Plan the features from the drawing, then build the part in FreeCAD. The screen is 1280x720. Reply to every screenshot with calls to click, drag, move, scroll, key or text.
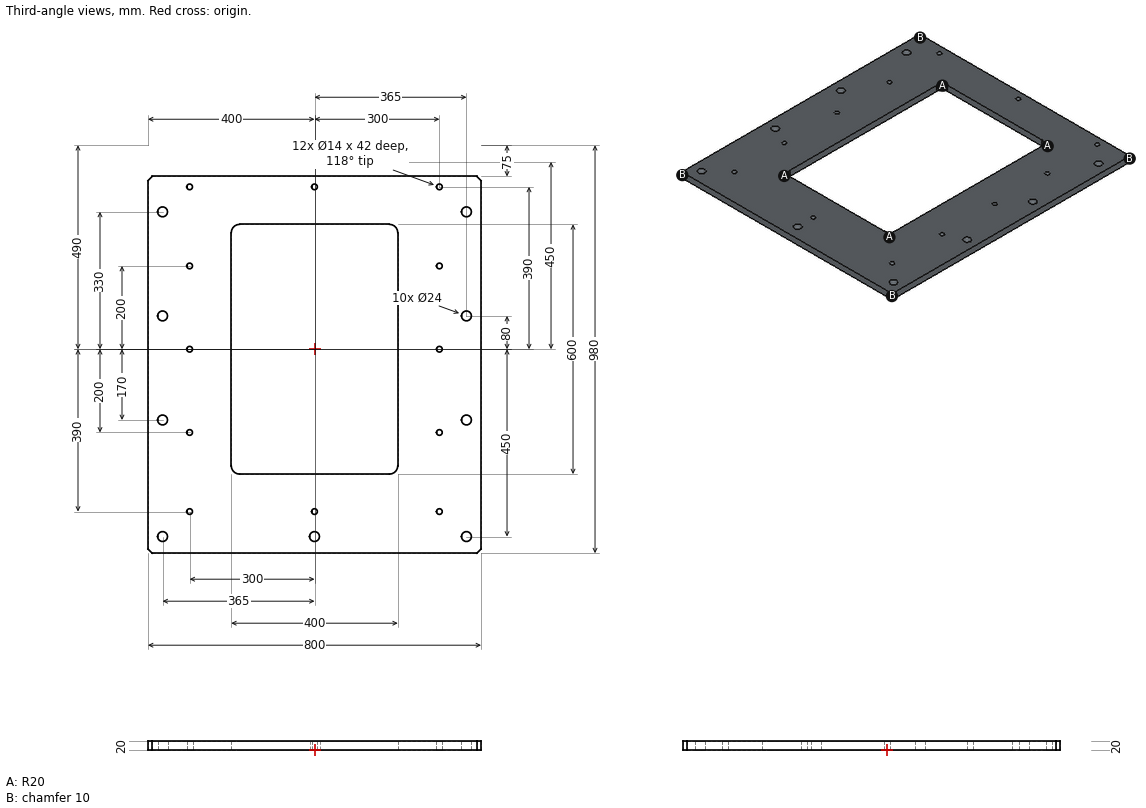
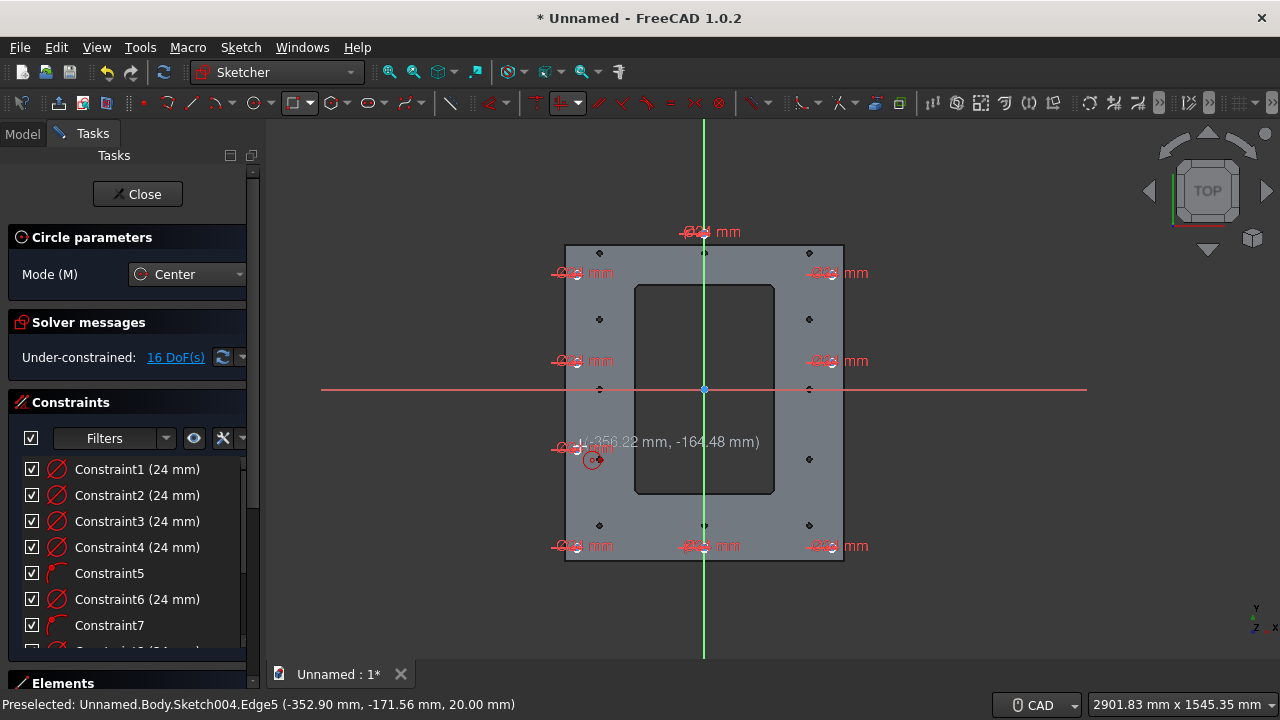
scroll(832, 449, up, 9)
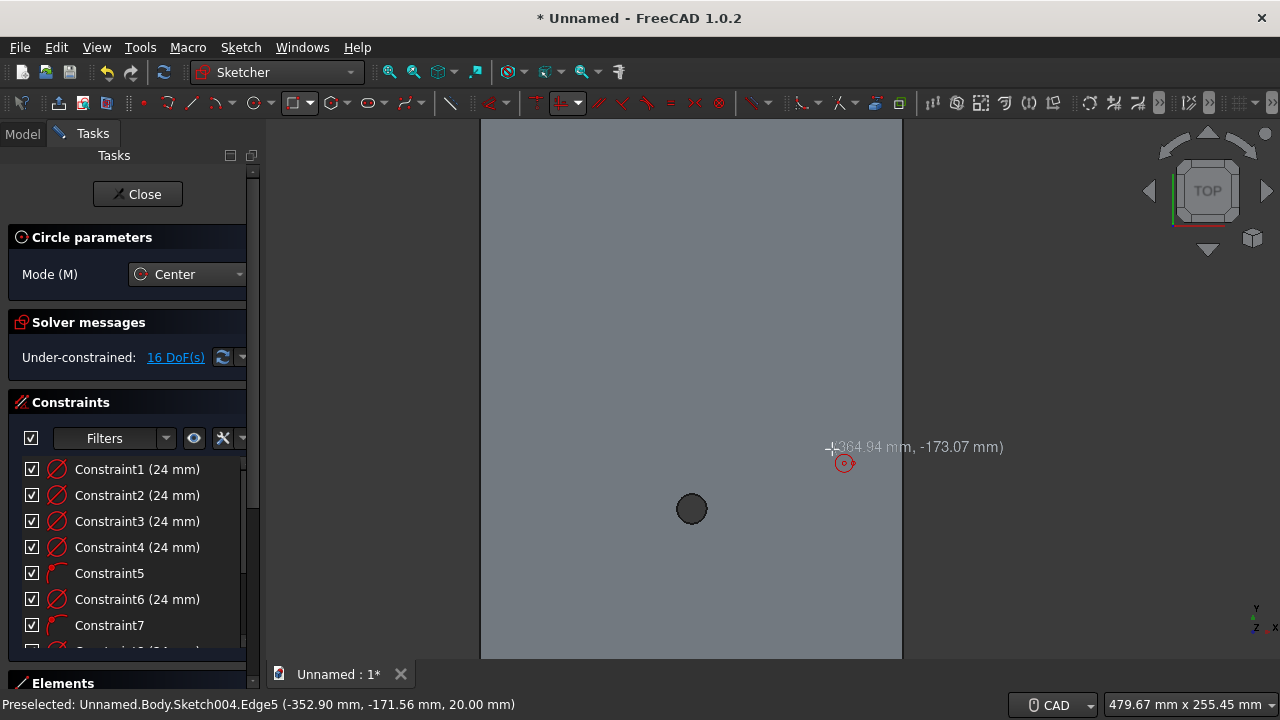
scroll(833, 449, down, 9)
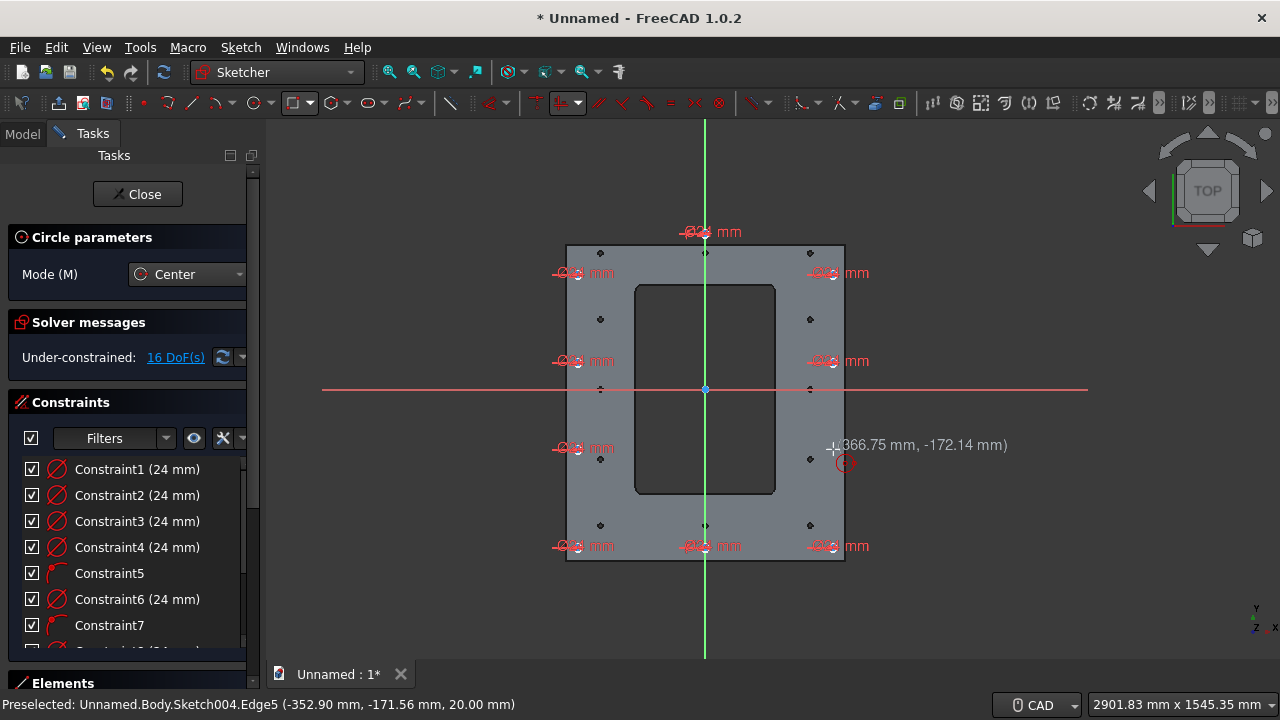
click(833, 449)
move(836, 446)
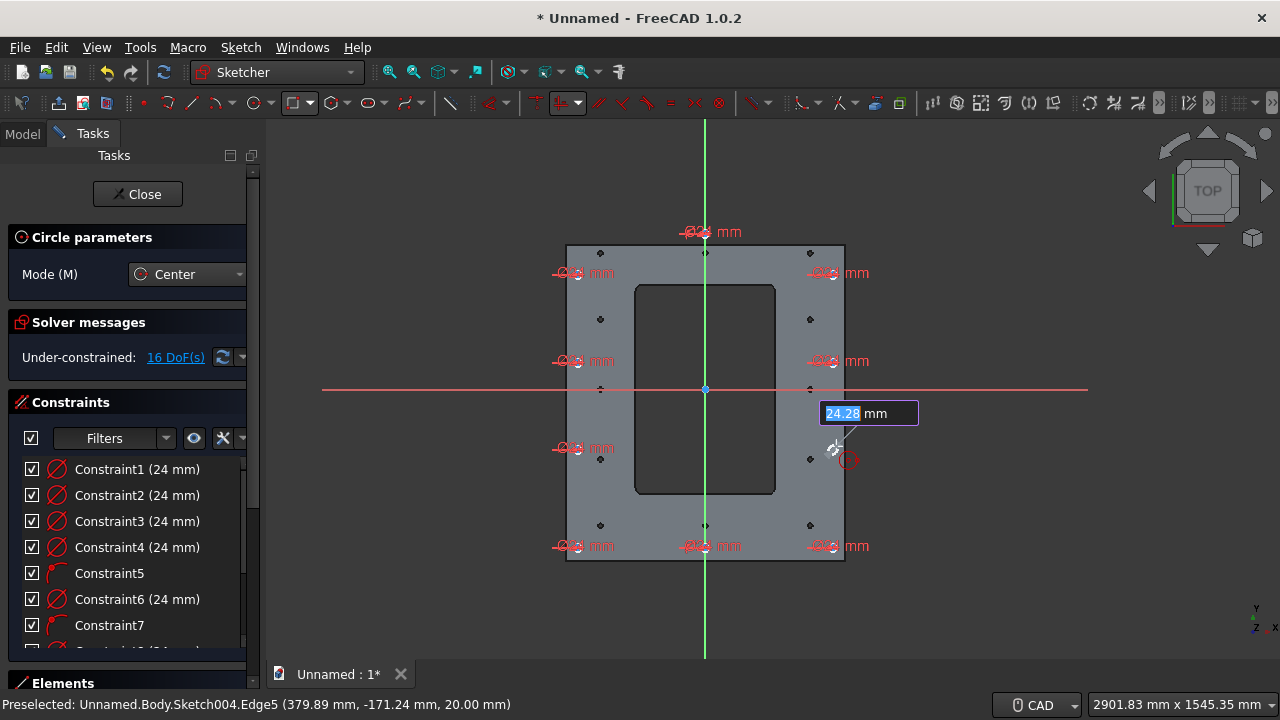
text(24)
key(Return)
key(Escape)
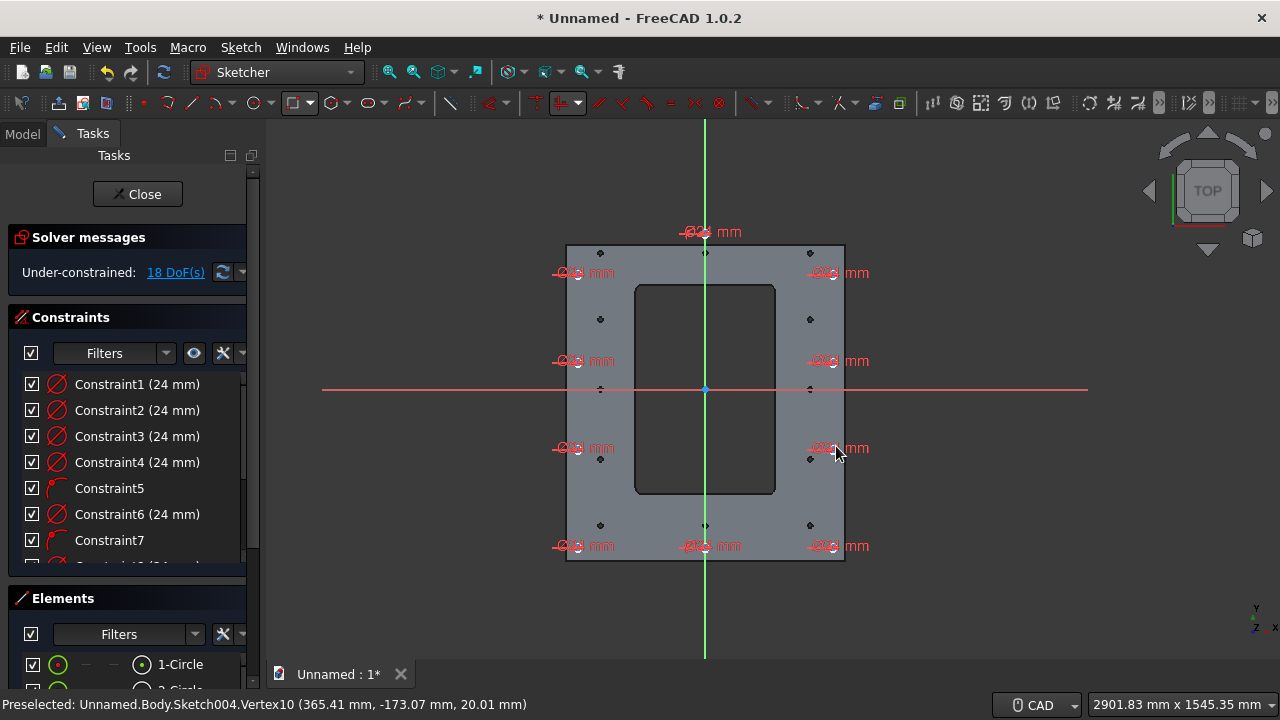
click(833, 363)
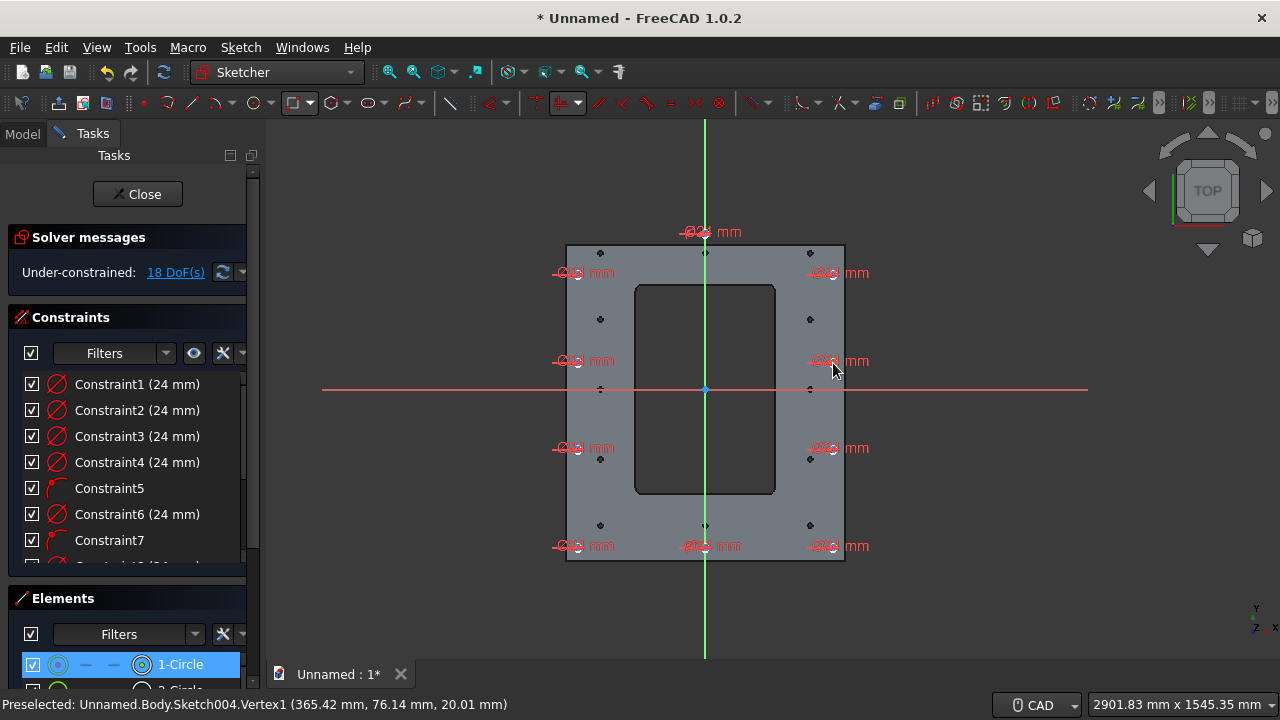
click(833, 548)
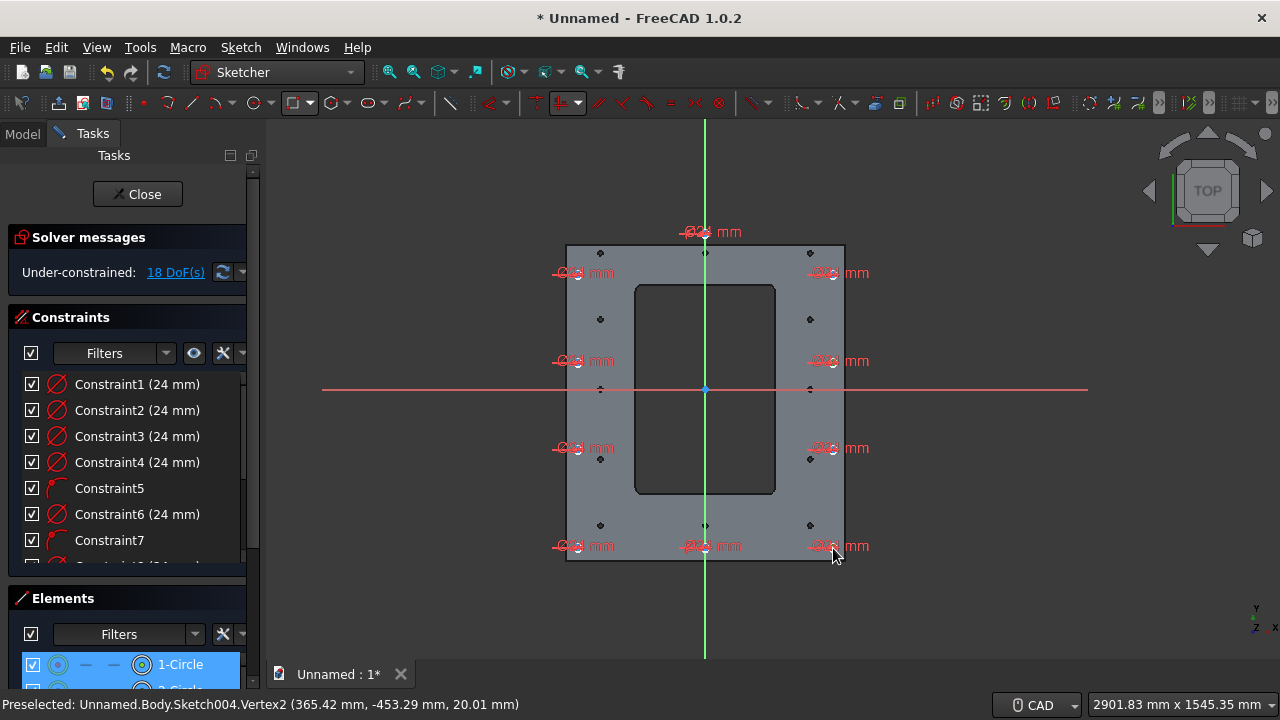
click(580, 104)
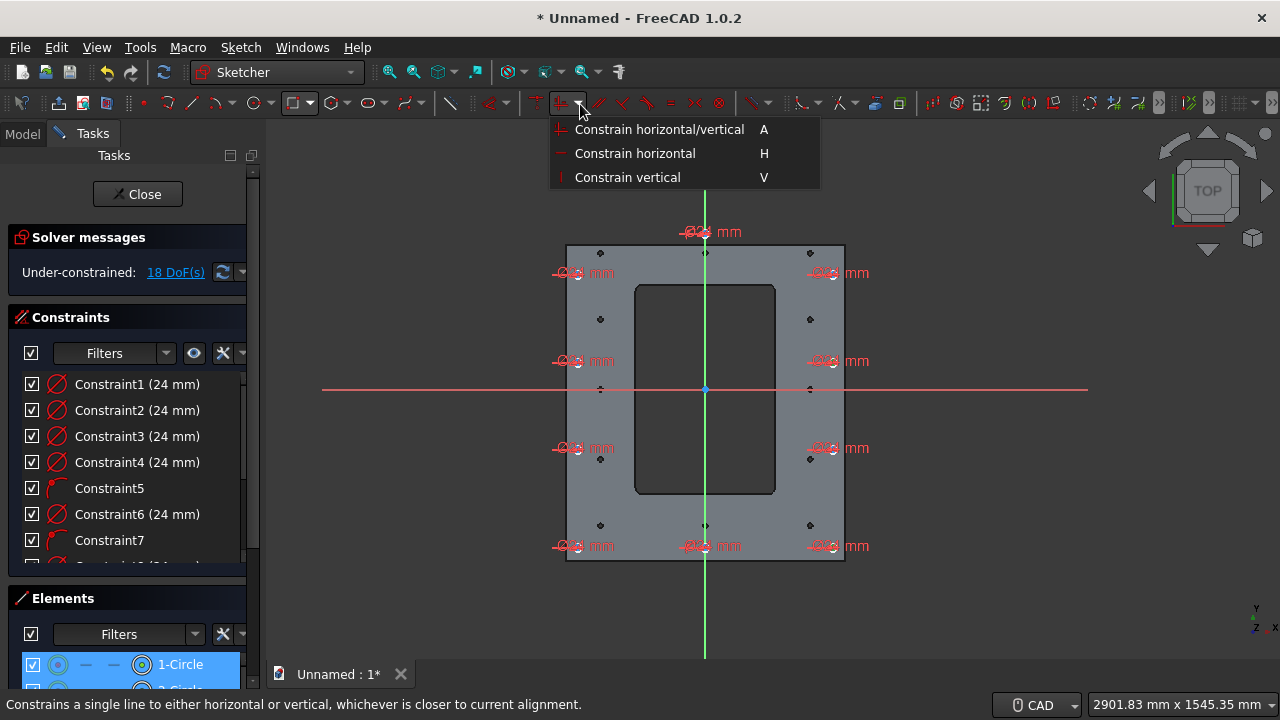
click(685, 177)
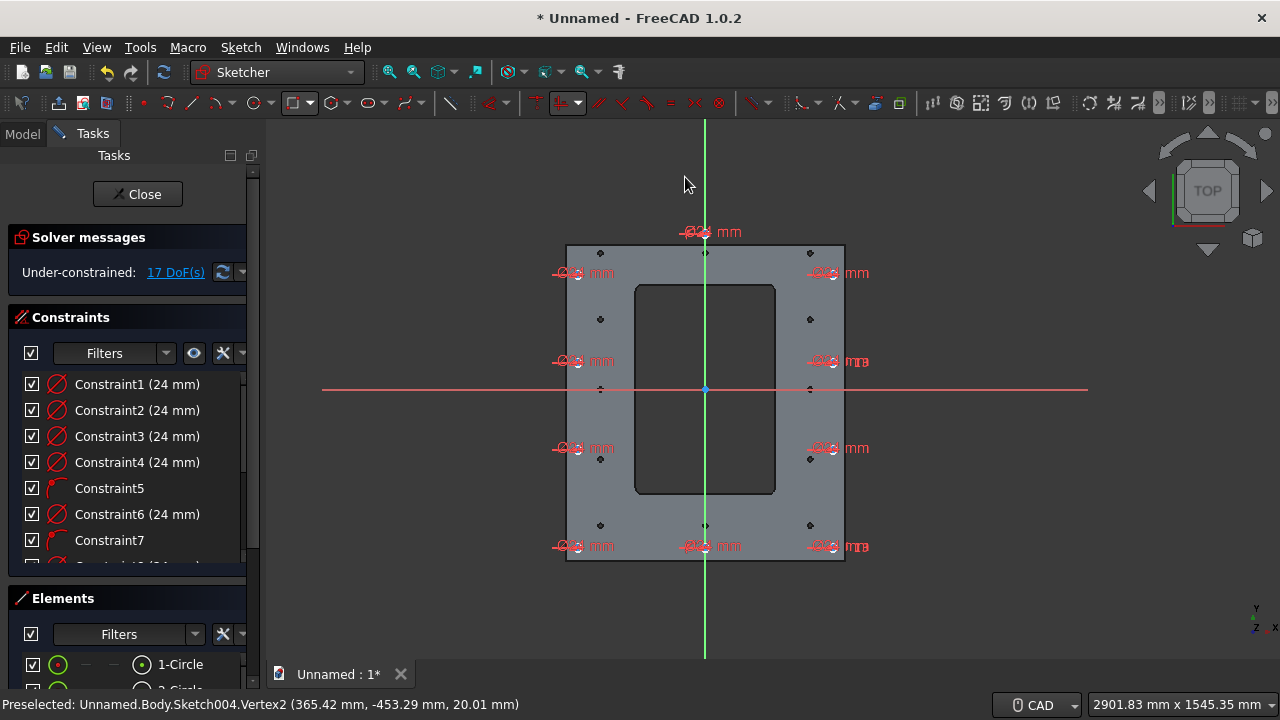
click(833, 548)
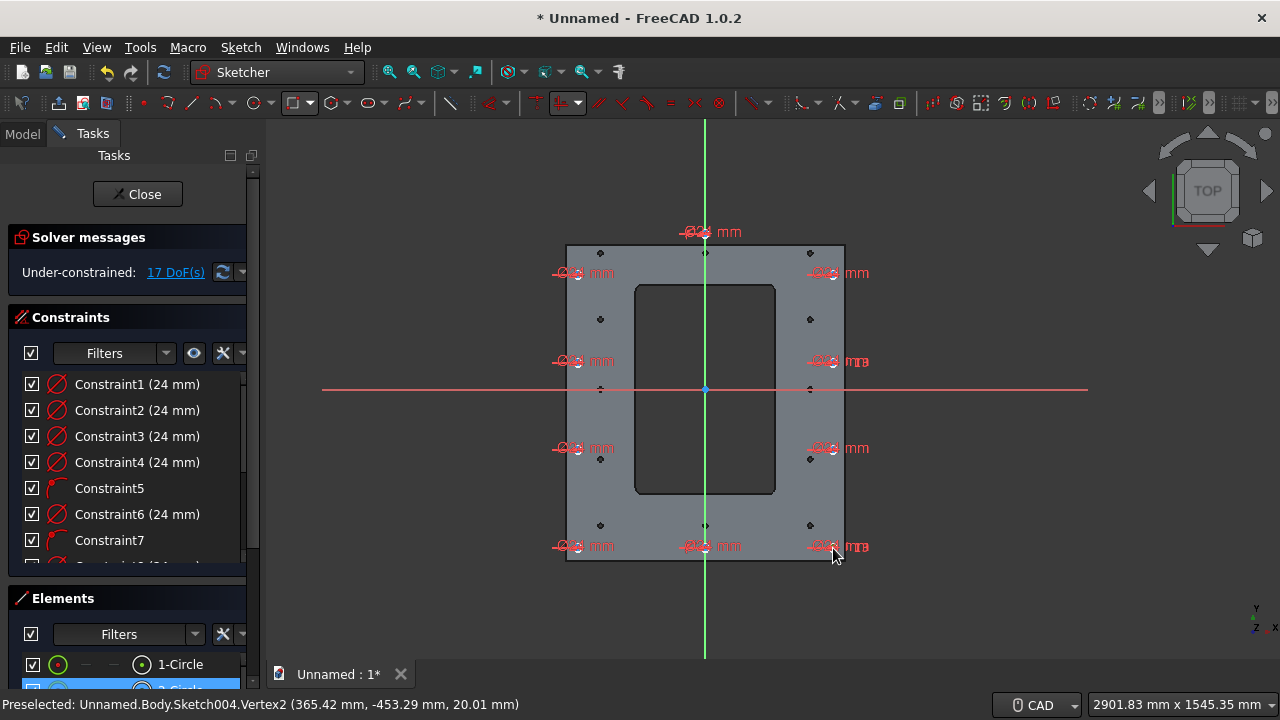
click(578, 548)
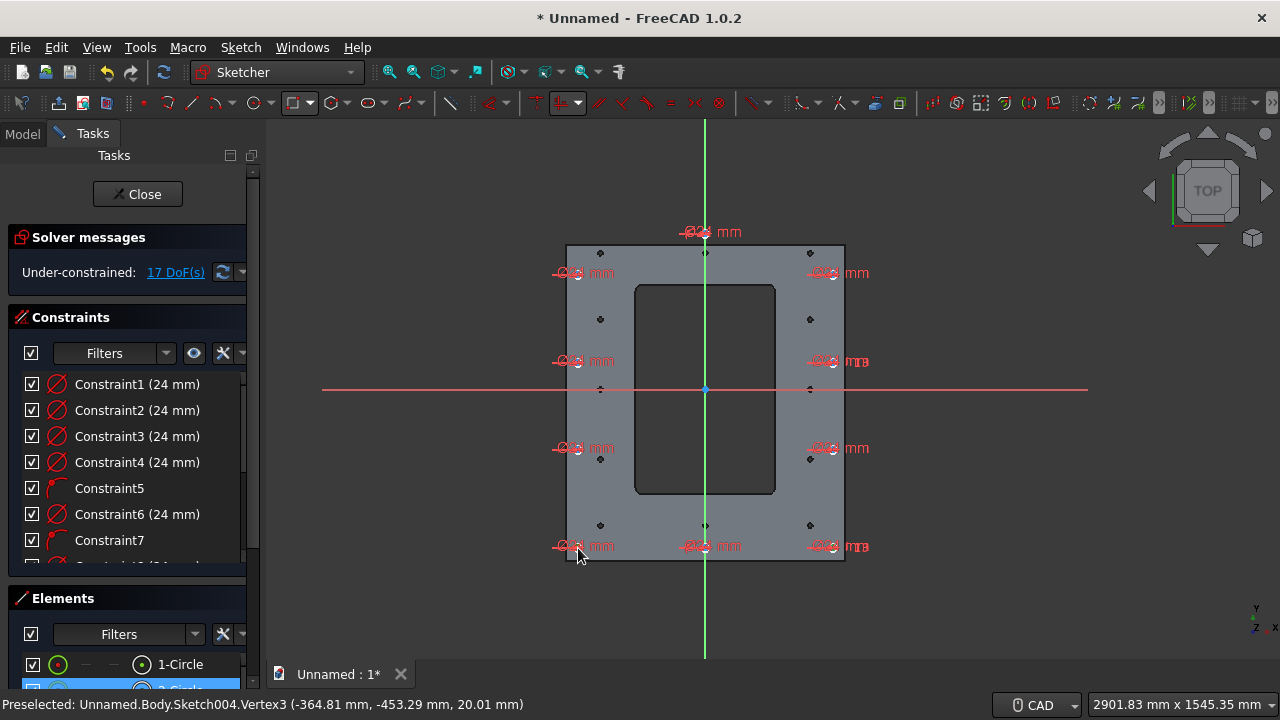
key(h)